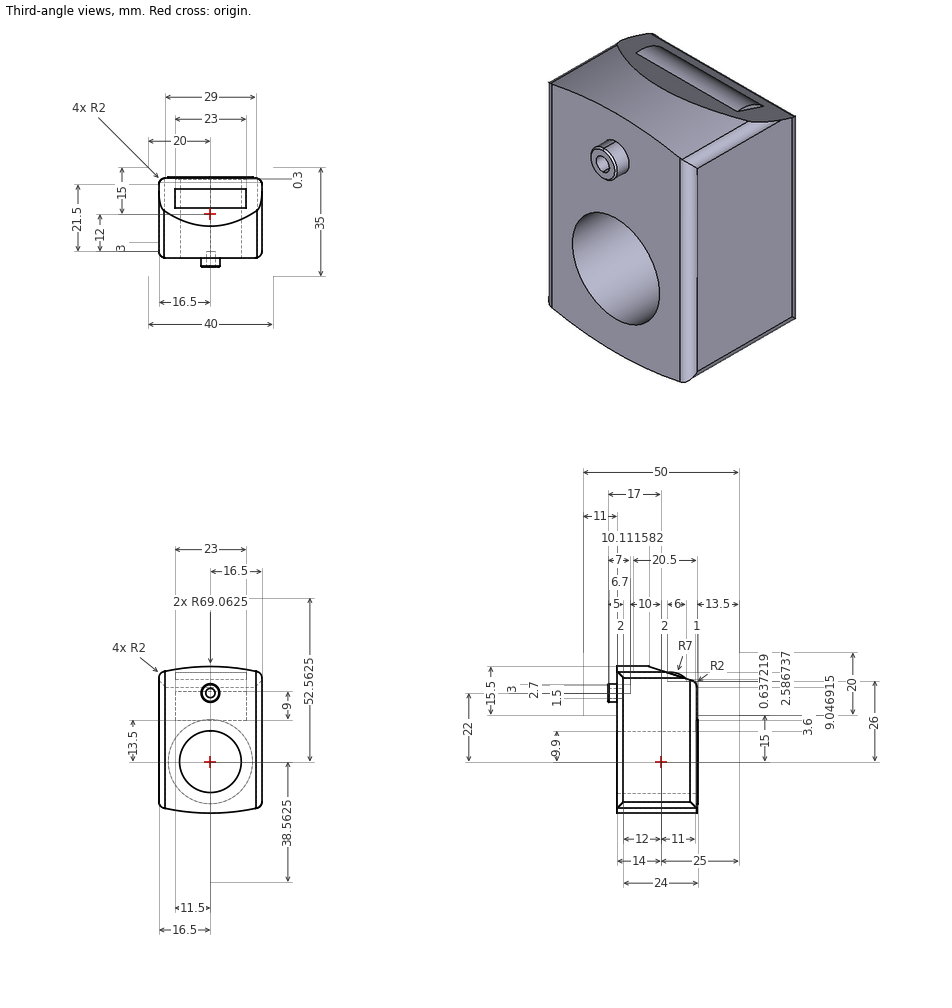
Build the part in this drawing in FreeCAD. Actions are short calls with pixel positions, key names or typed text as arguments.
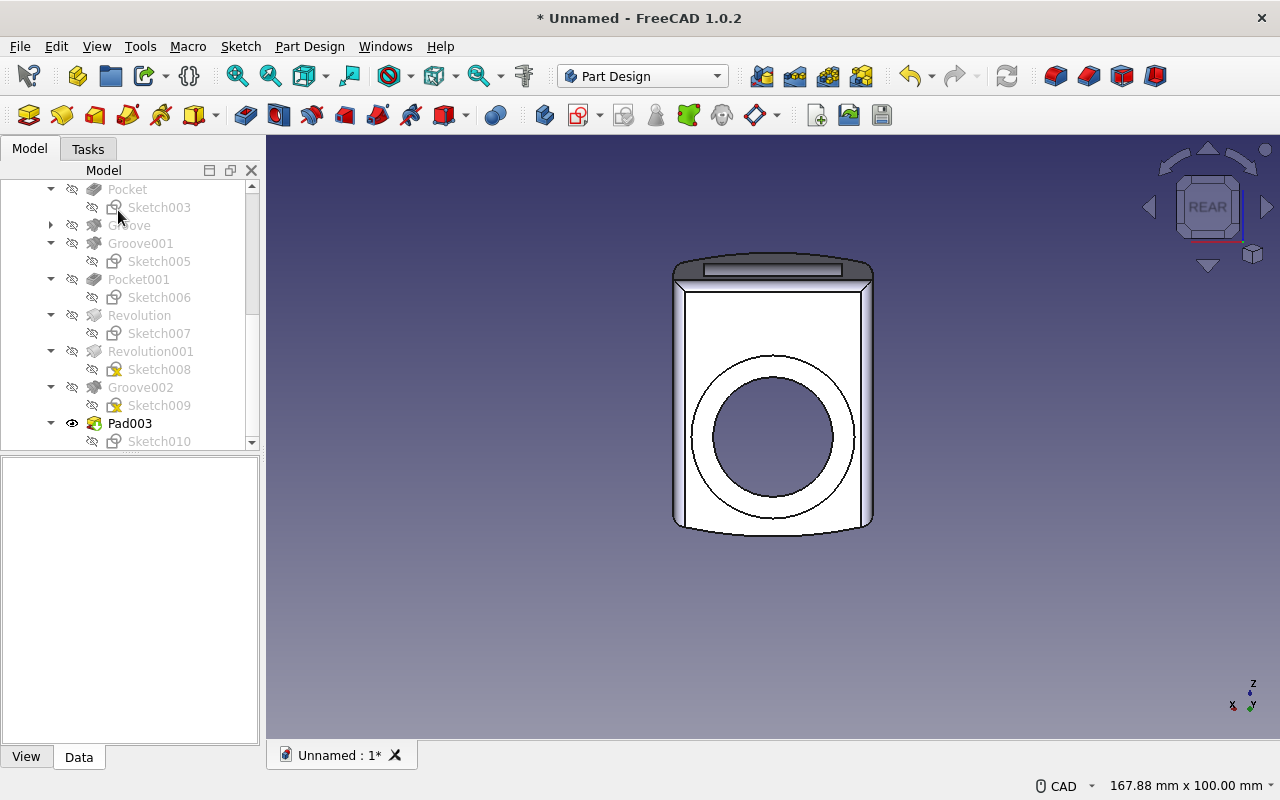
click(723, 343)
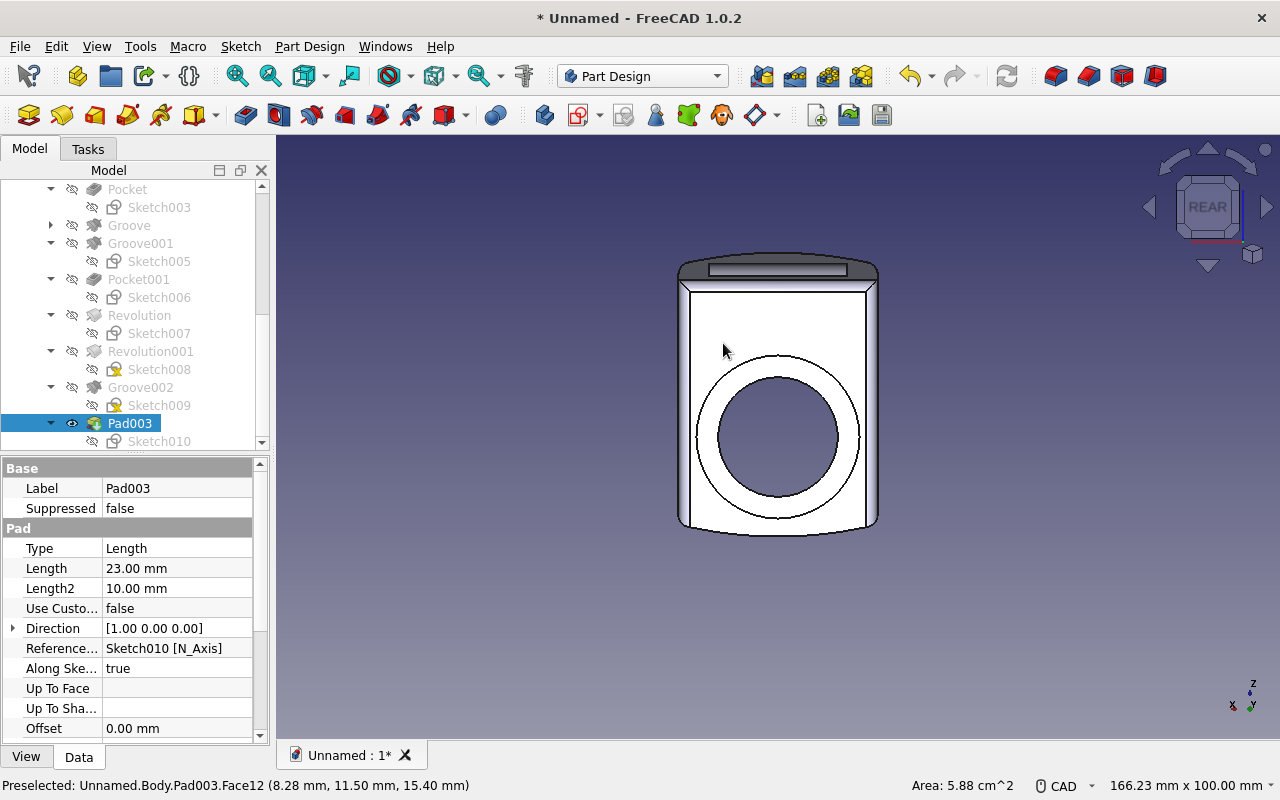
click(578, 116)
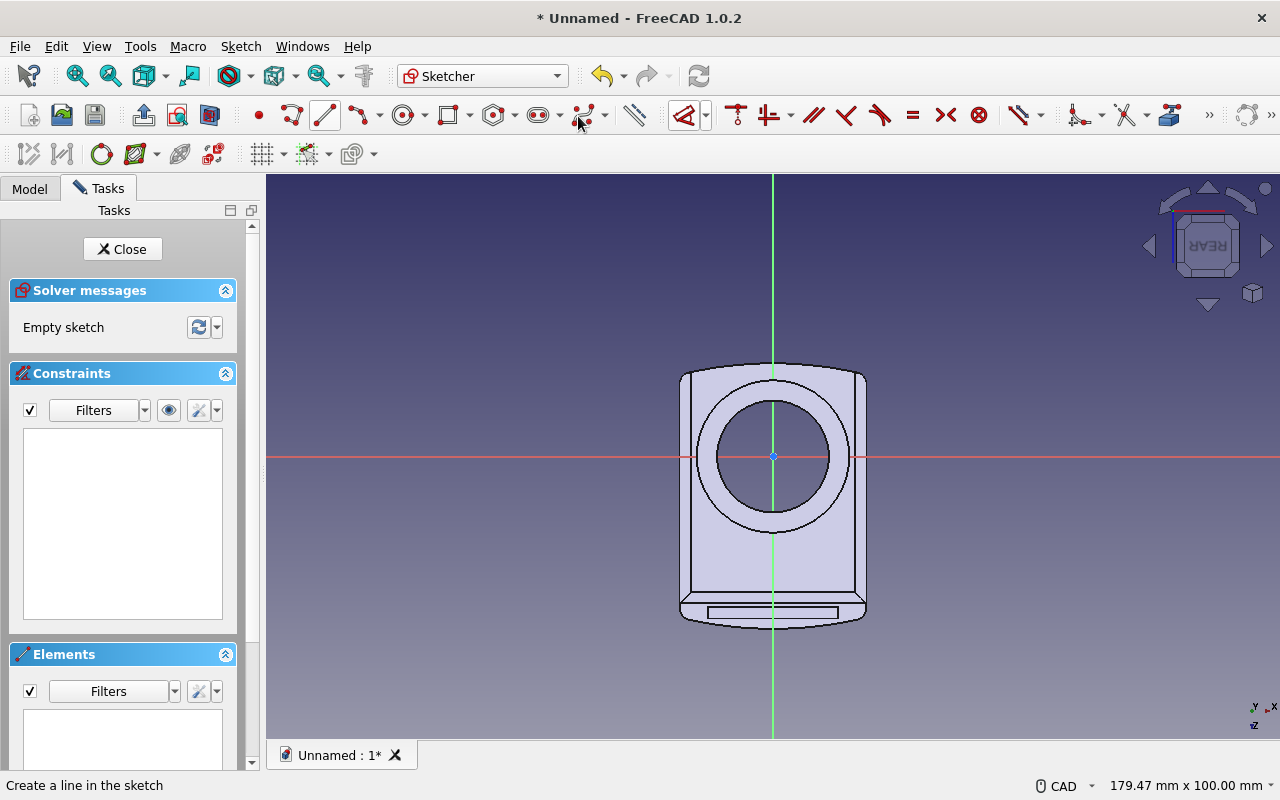
scroll(813, 557, up, 5)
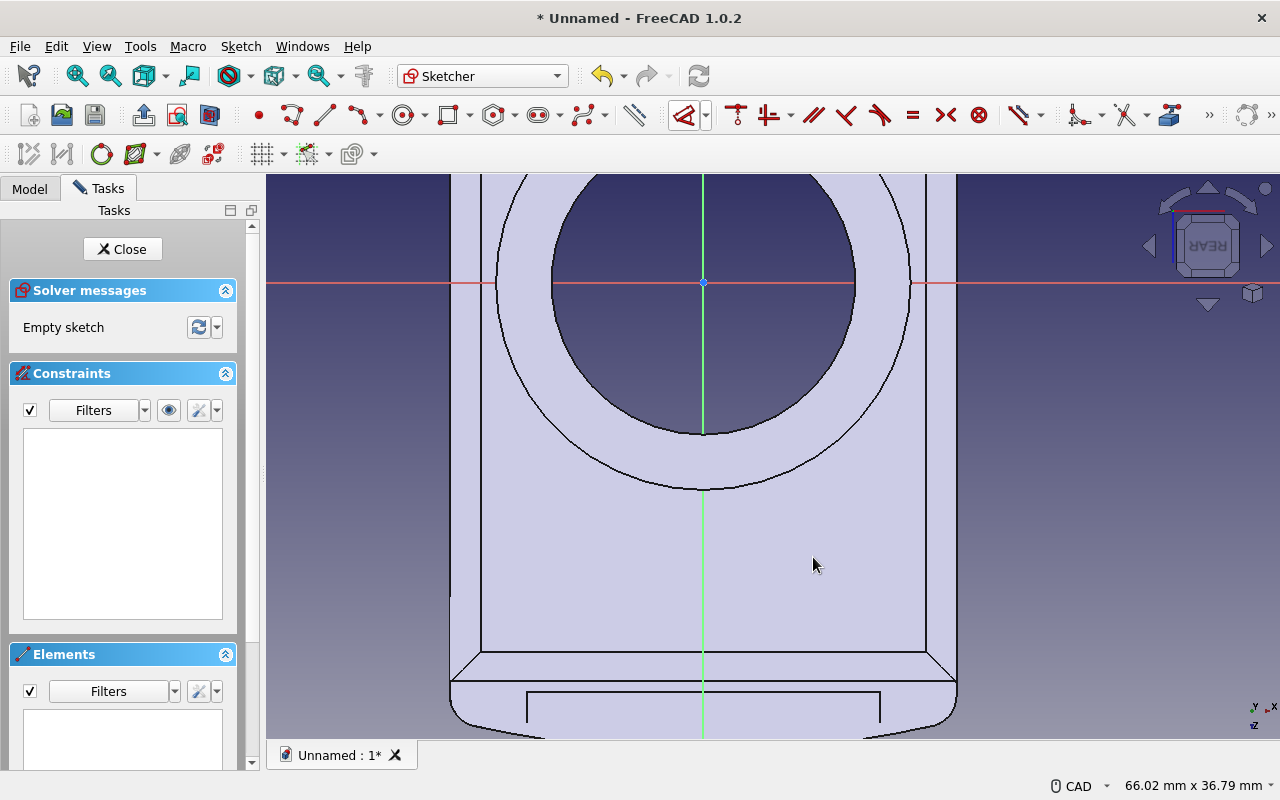
click(448, 116)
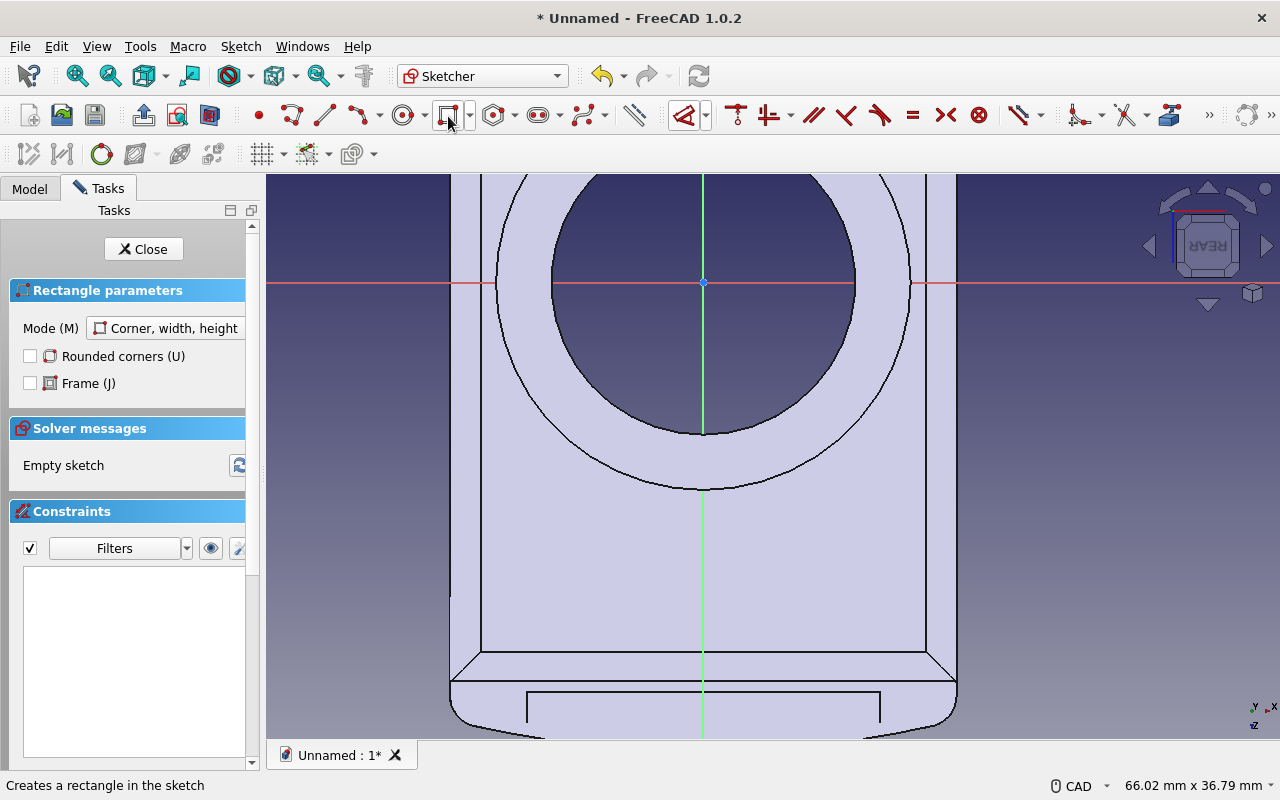
click(527, 490)
move(880, 628)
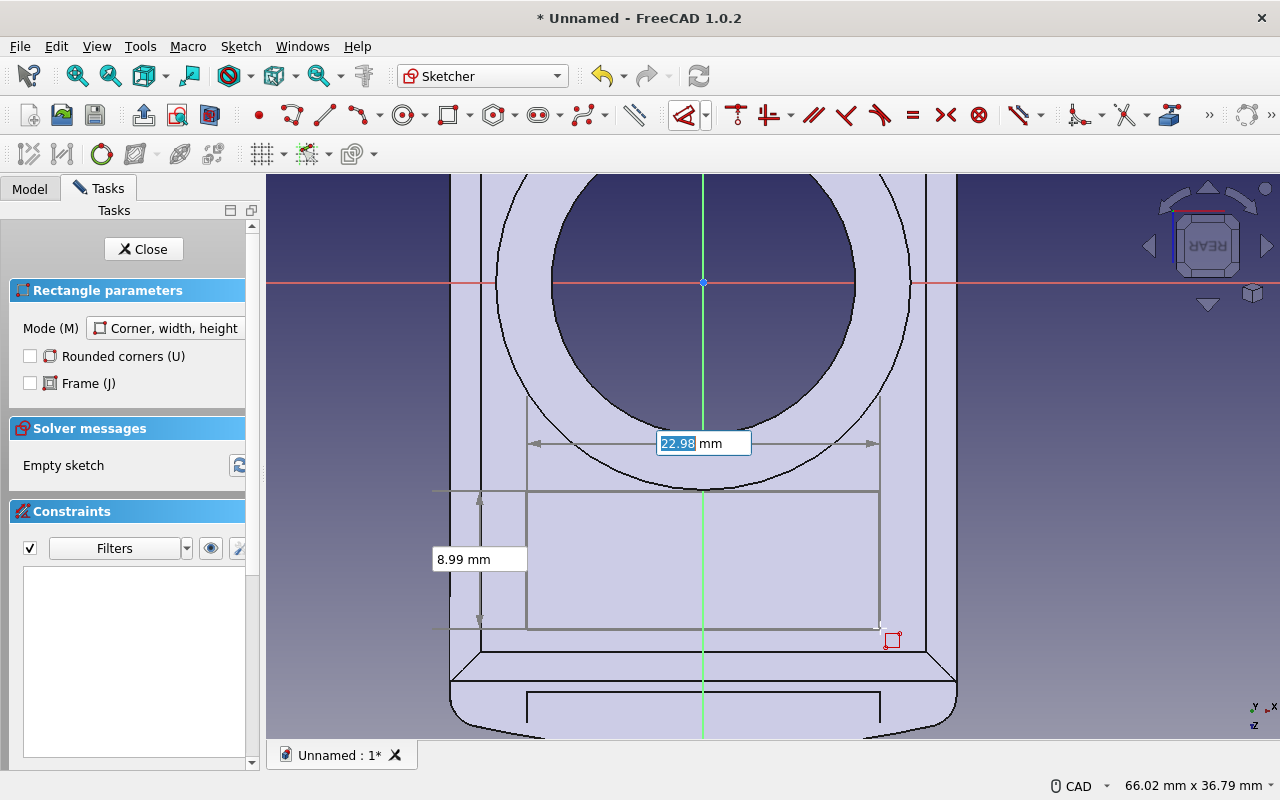
text(23)
key(Tab)
text(9)
key(Return)
key(Escape)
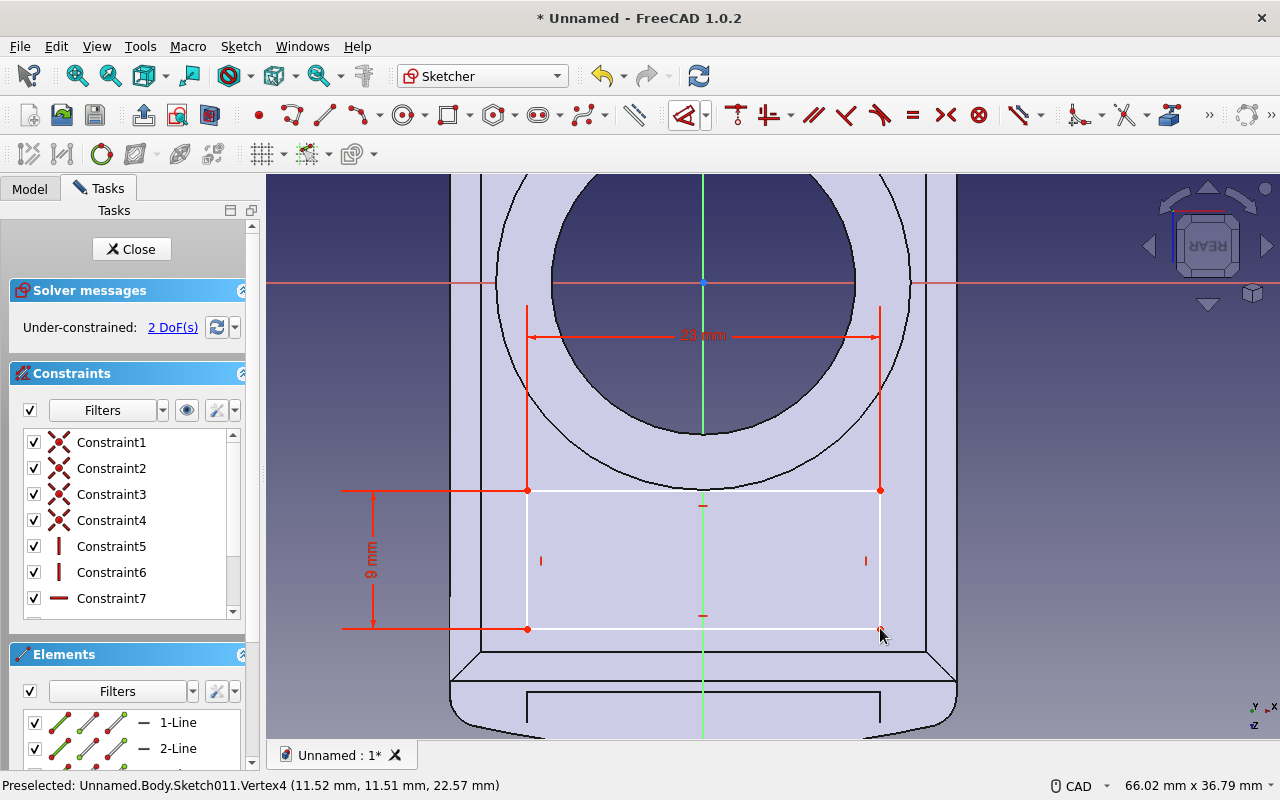
click(527, 491)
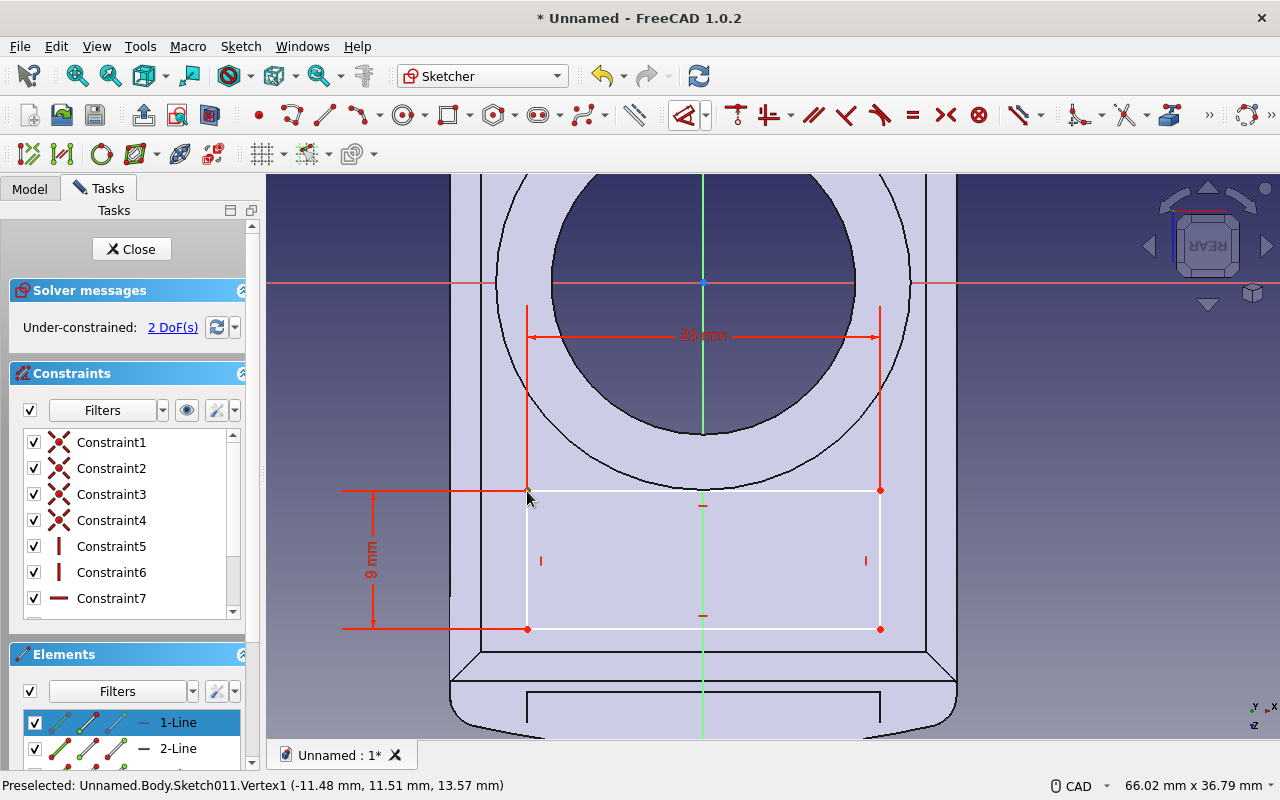
click(706, 116)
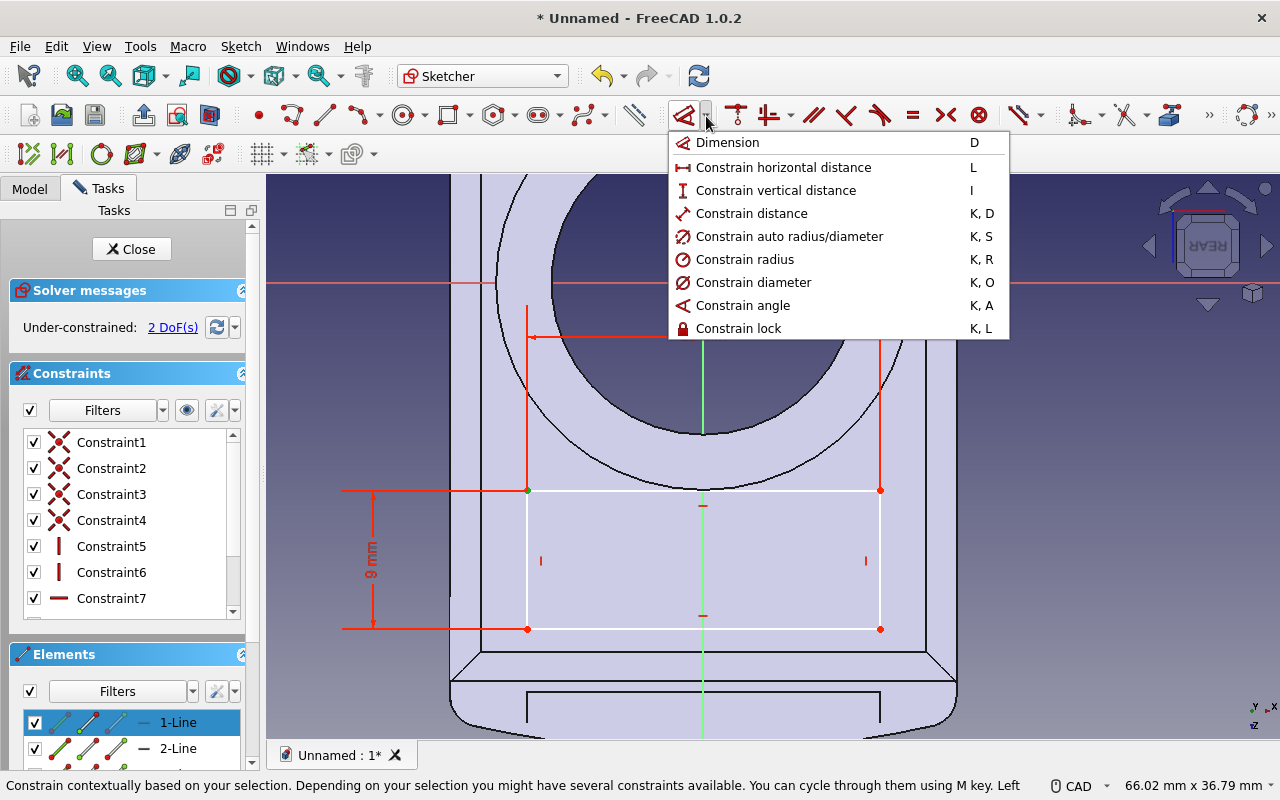
click(839, 168)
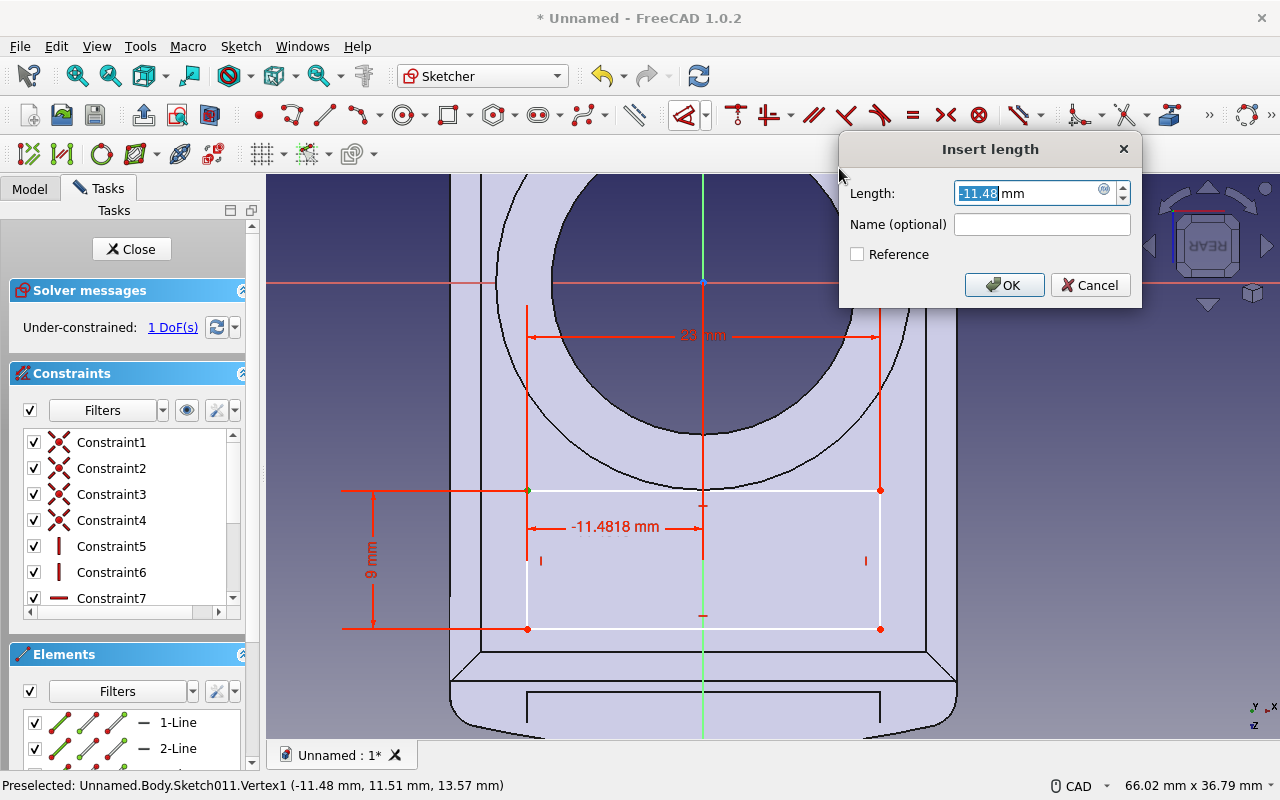
text(-11.5)
key(Return)